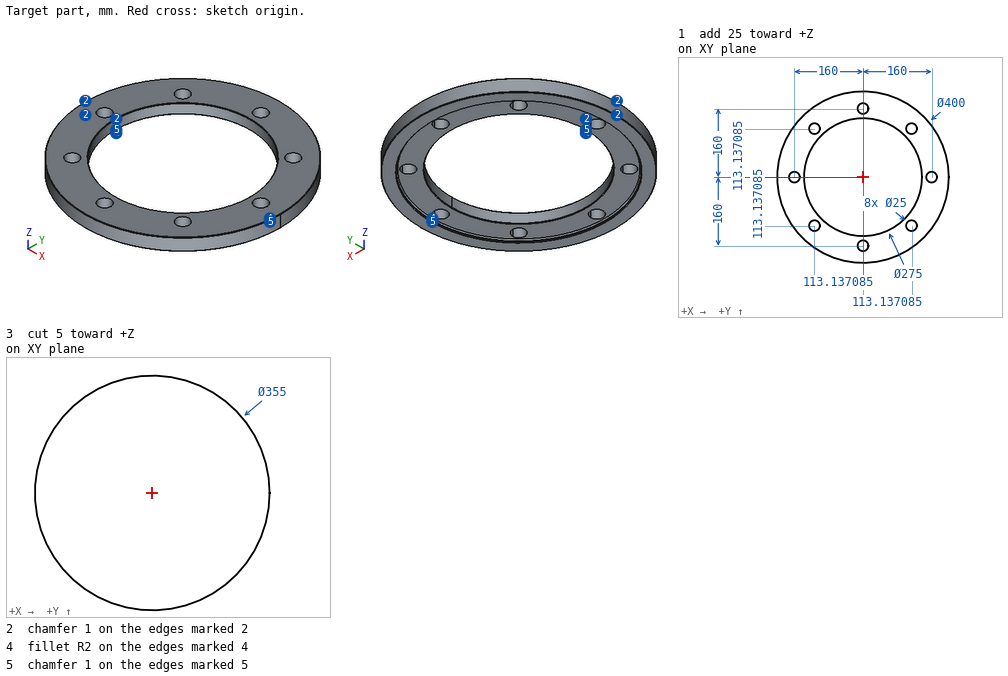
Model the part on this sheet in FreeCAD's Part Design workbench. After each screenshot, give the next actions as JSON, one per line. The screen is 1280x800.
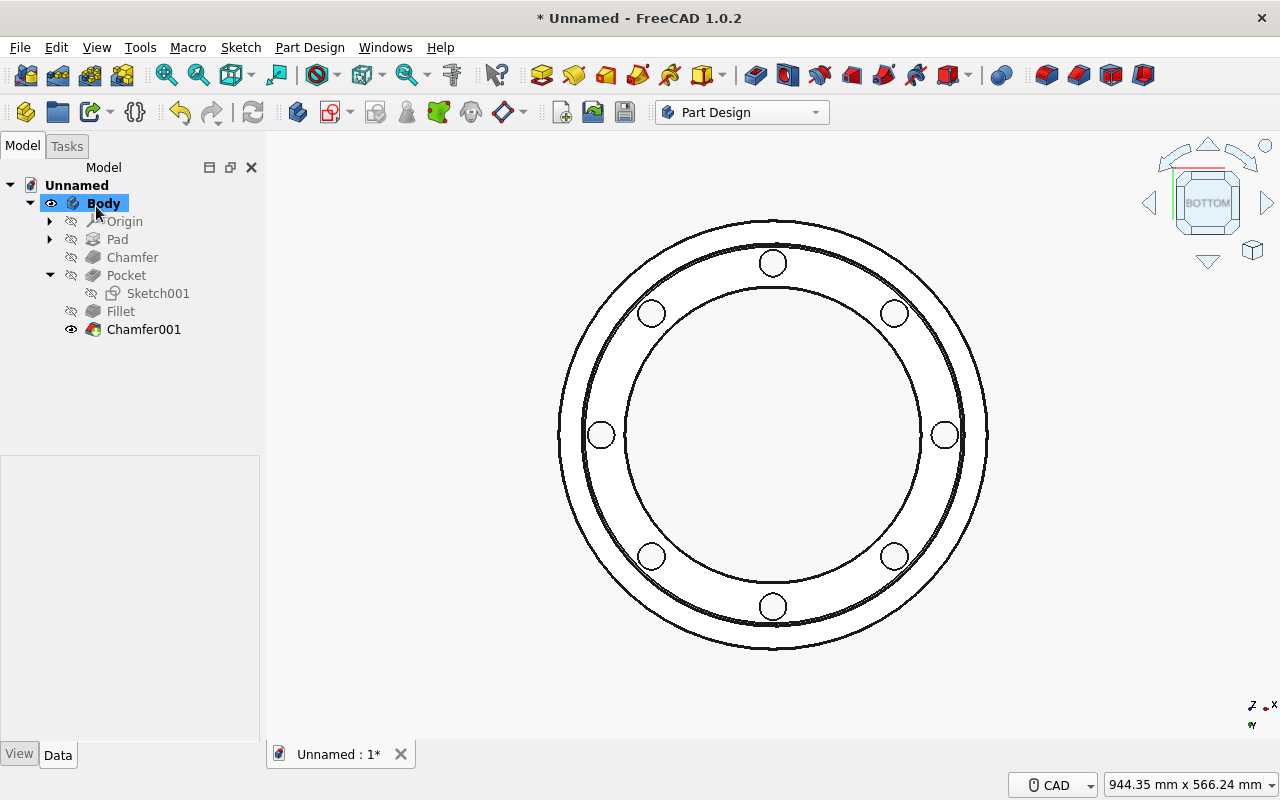
{"action": "key", "text": "0"}